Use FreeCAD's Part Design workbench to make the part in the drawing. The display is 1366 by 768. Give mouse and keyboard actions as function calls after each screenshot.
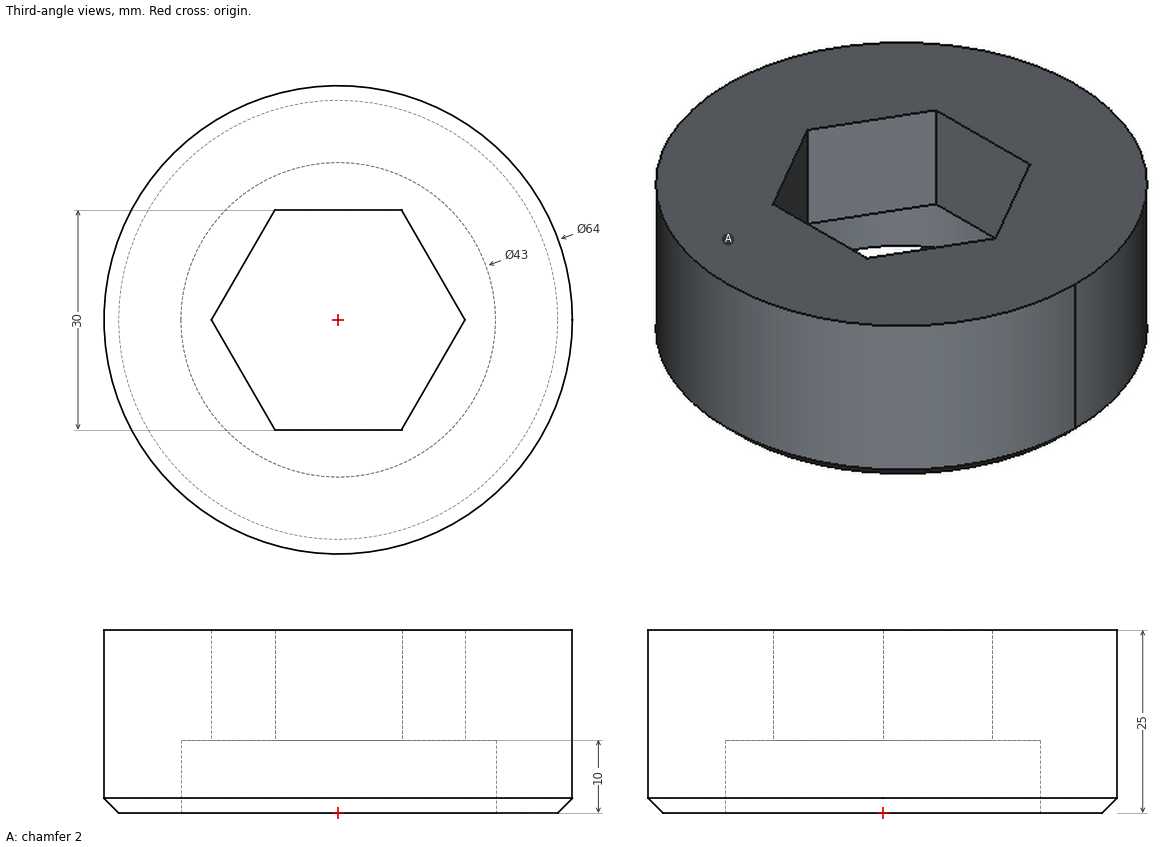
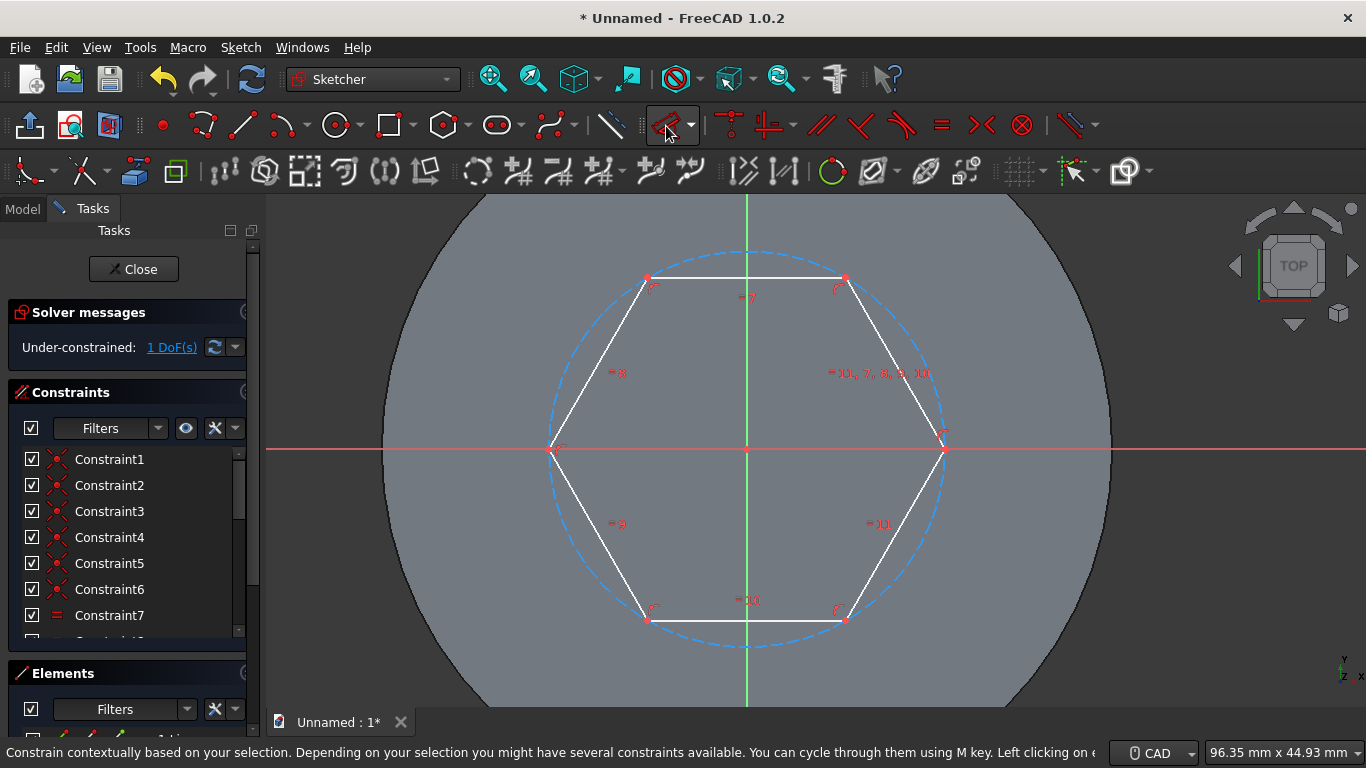
click(648, 621)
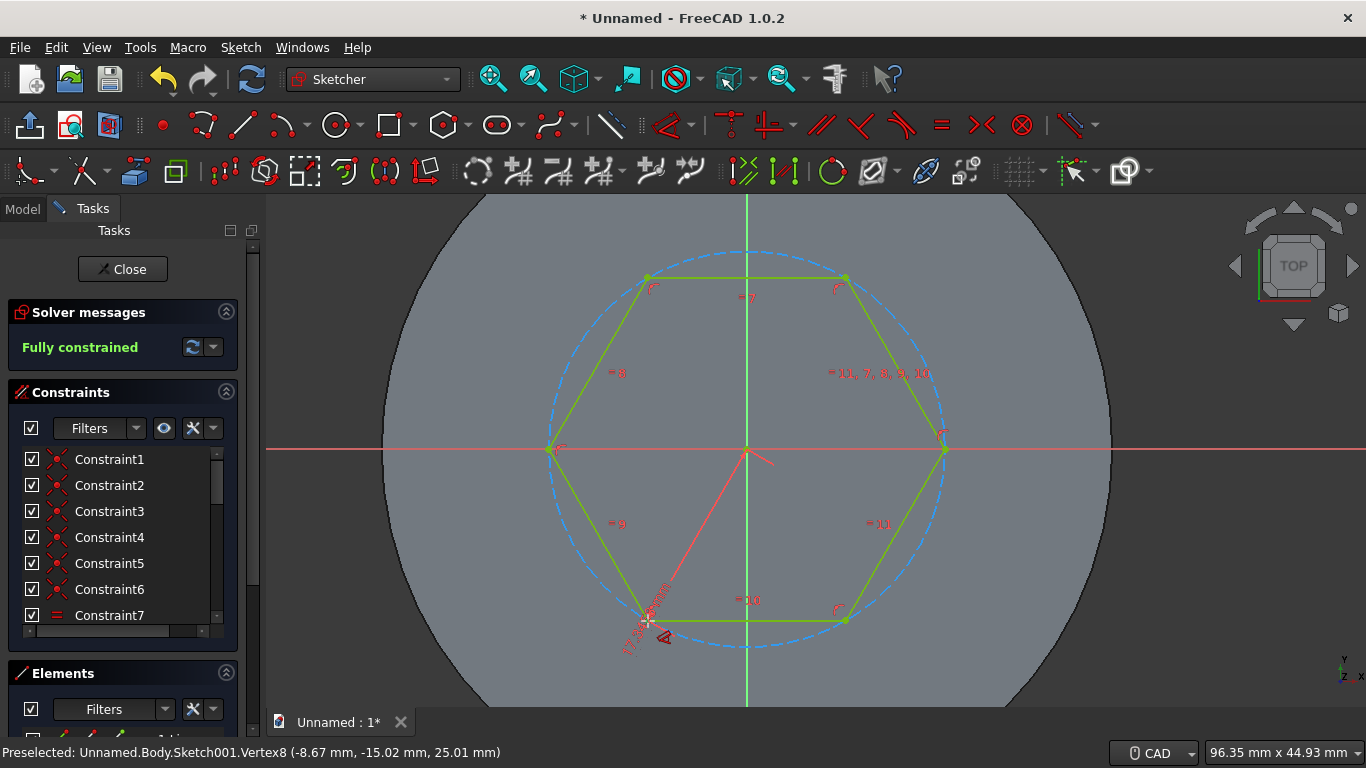
click(846, 278)
click(880, 370)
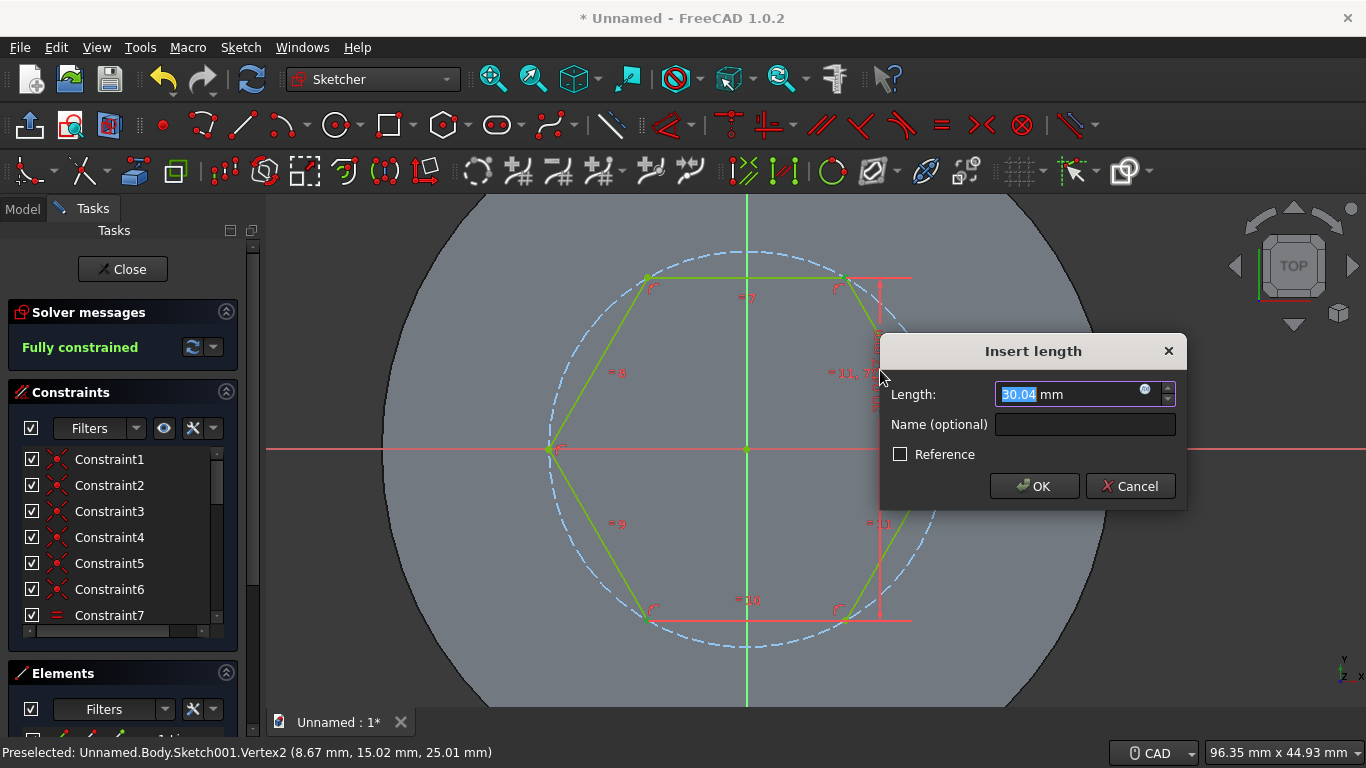
text(30)
key(Return)
key(Escape)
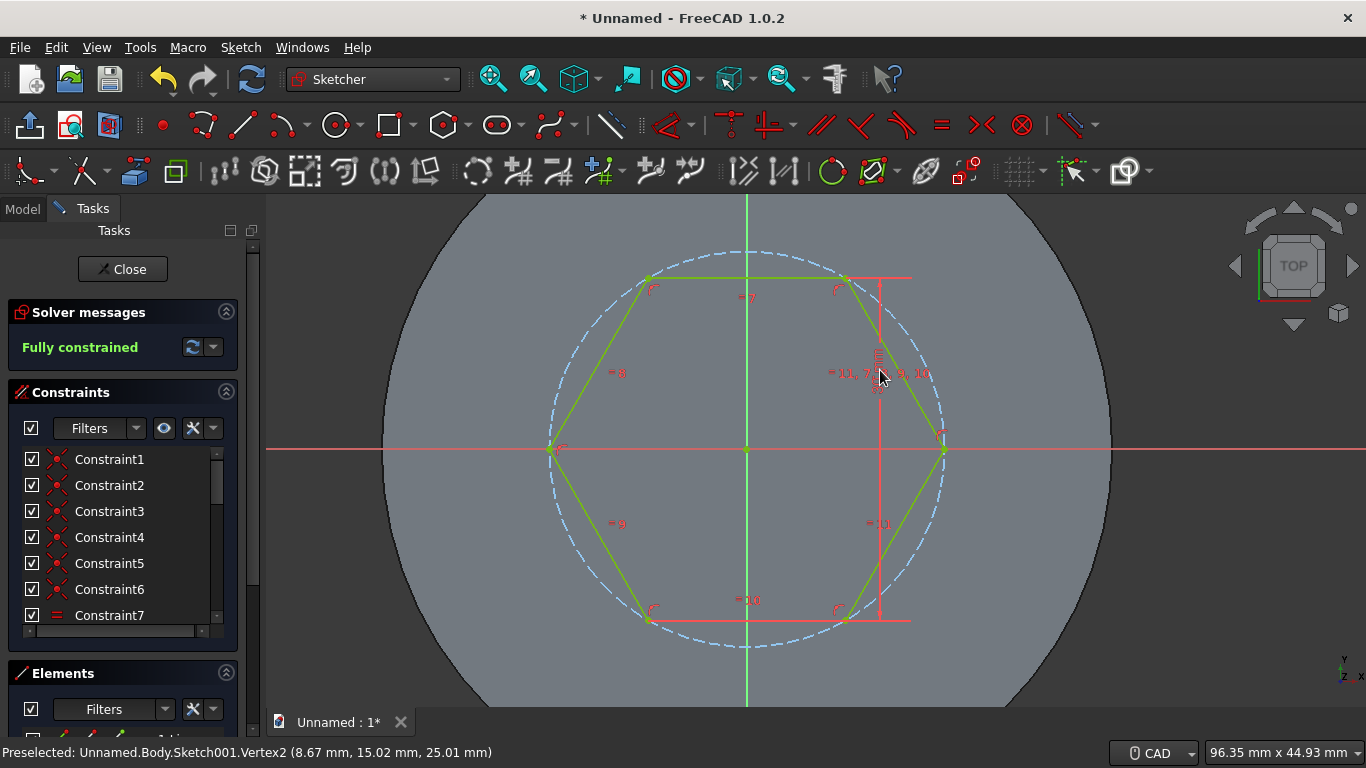
click(123, 269)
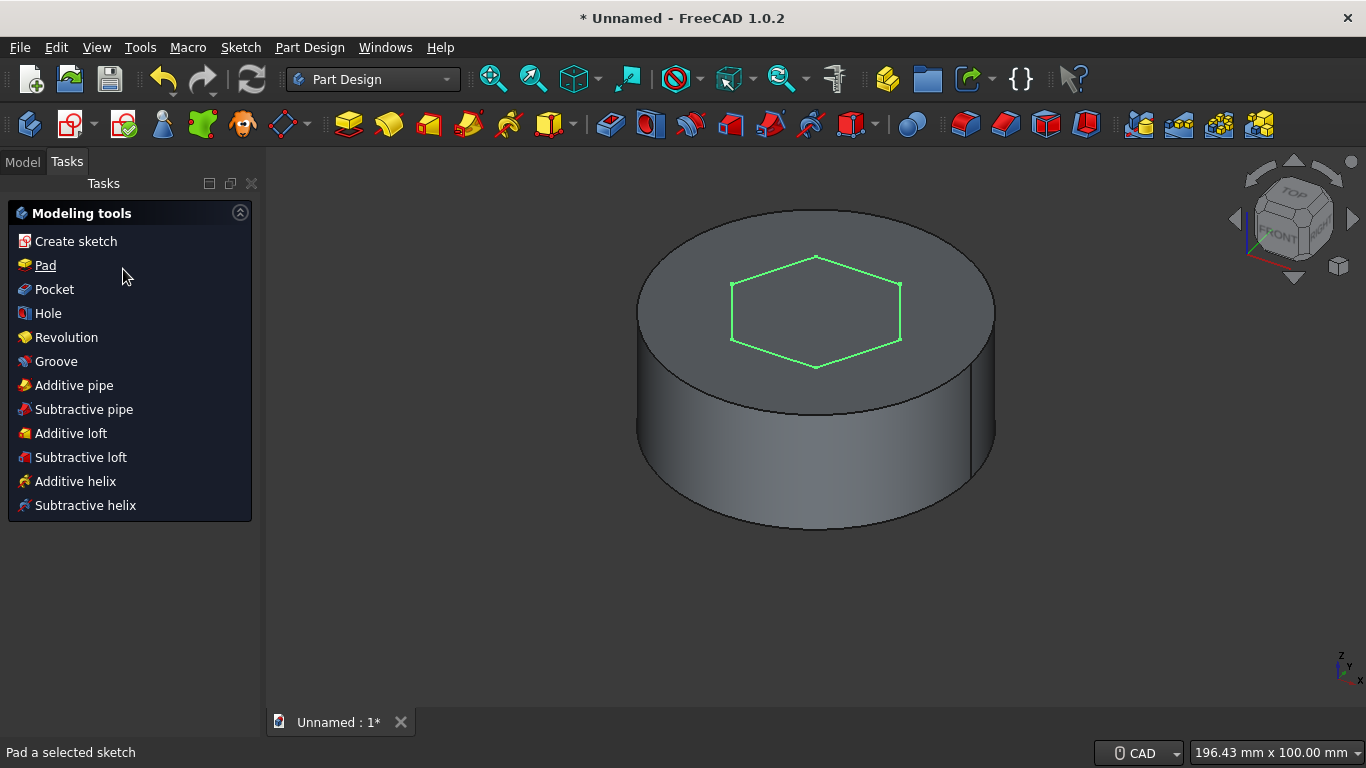
click(612, 124)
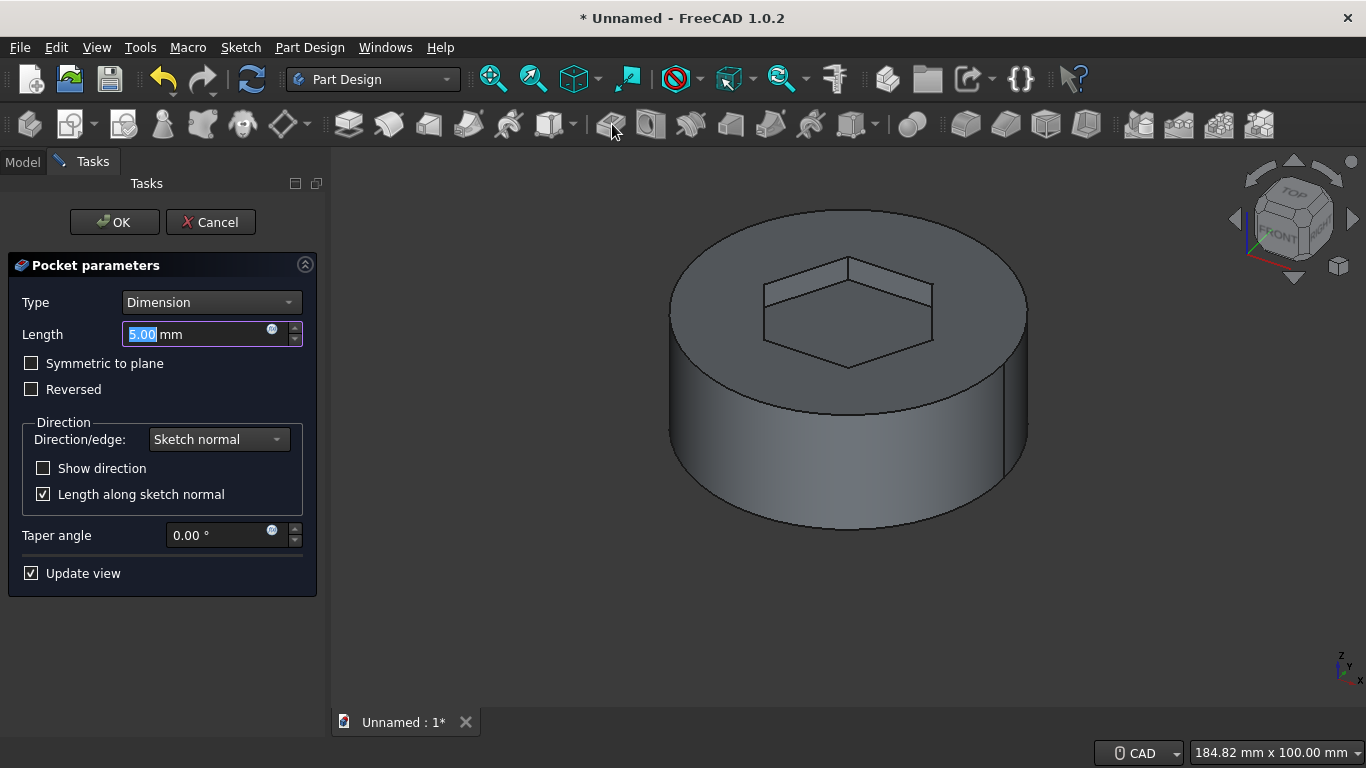
click(212, 302)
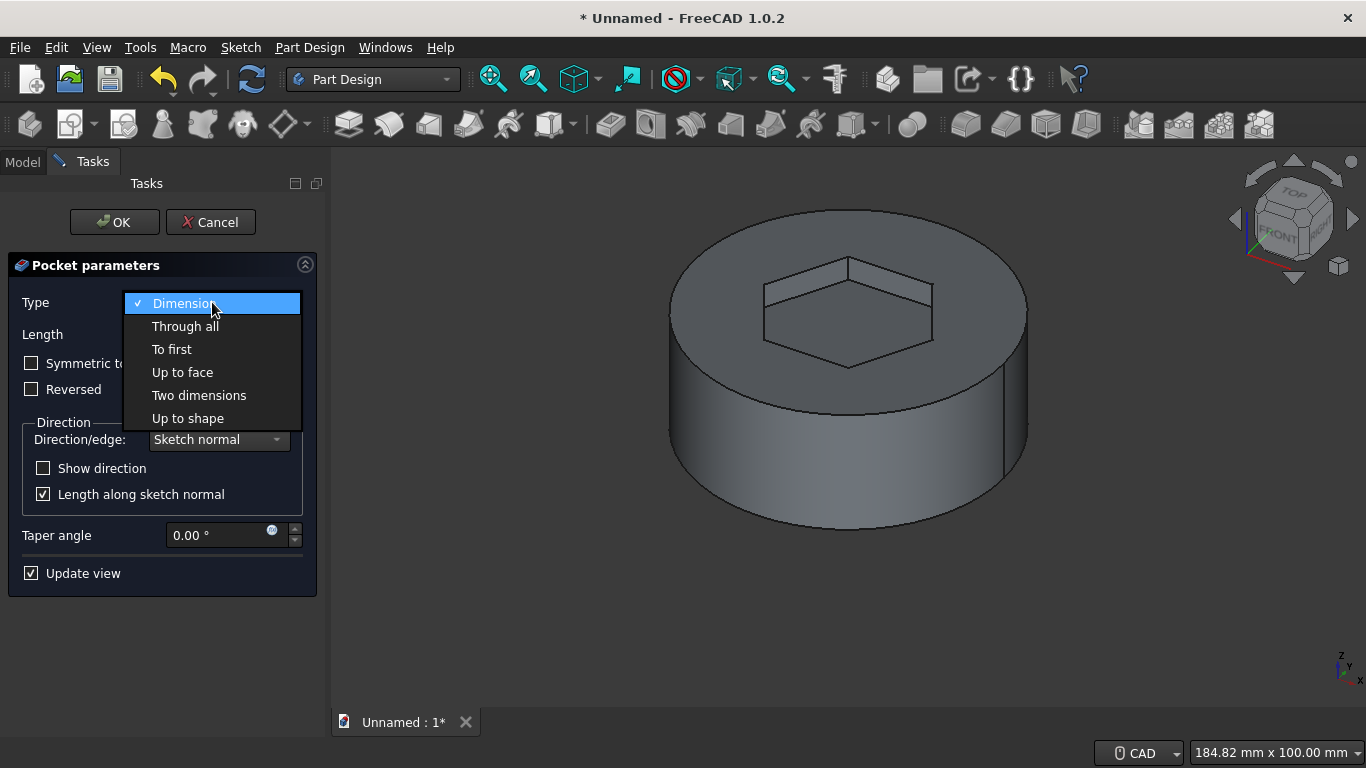
click(212, 326)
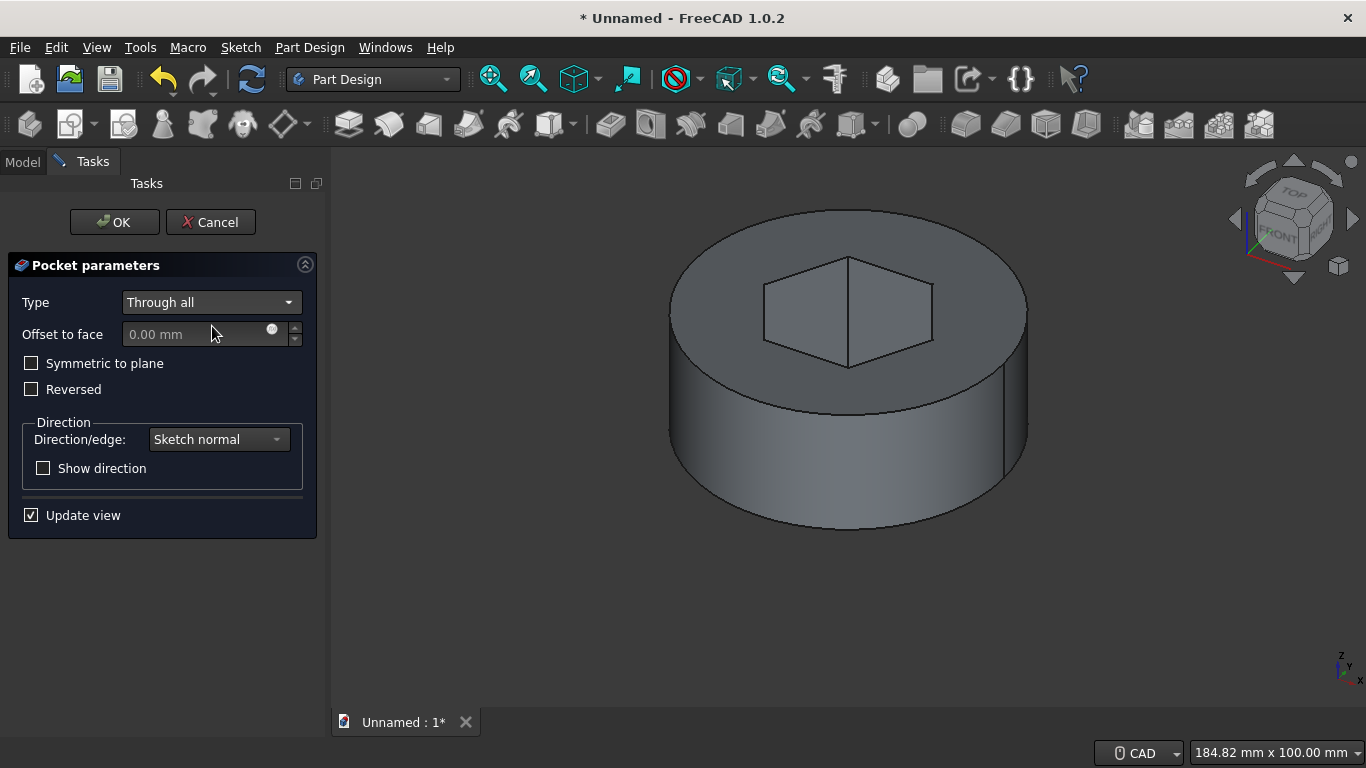
click(115, 222)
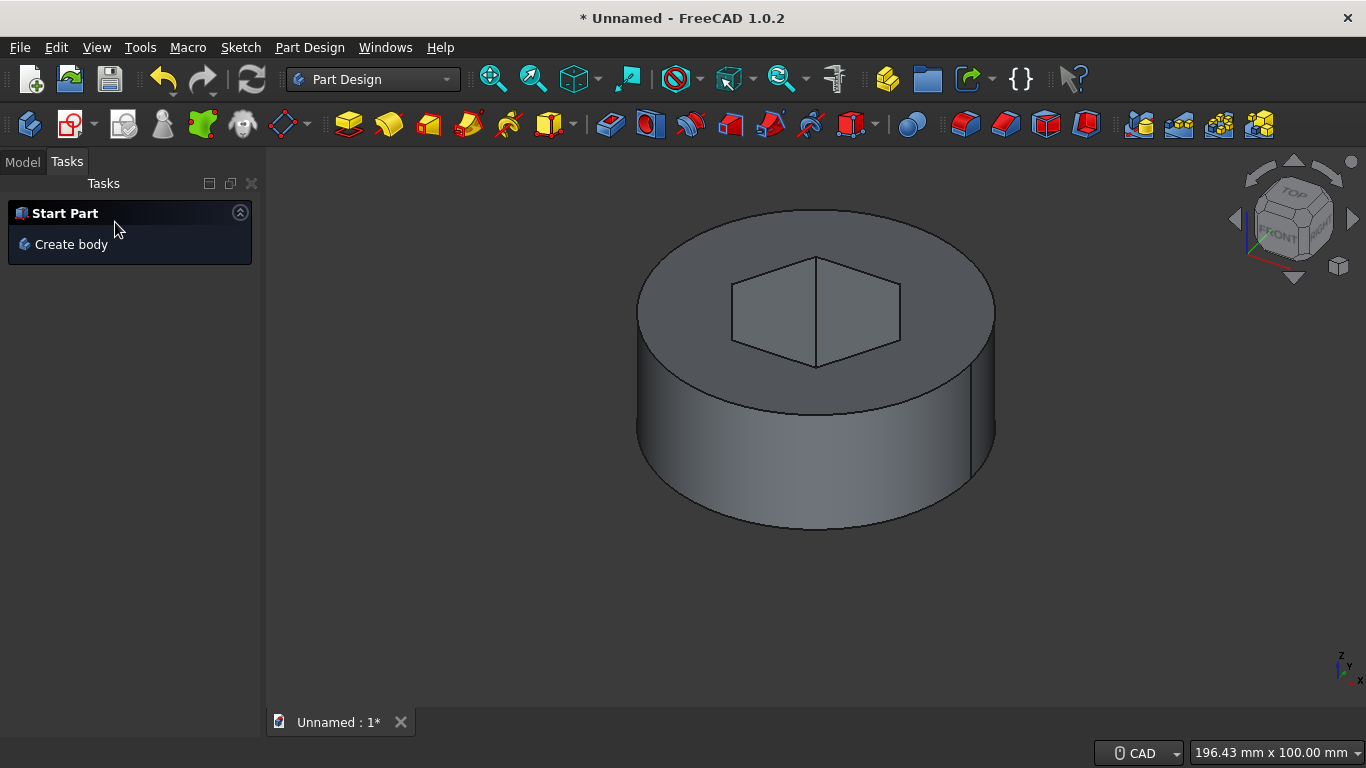
click(70, 124)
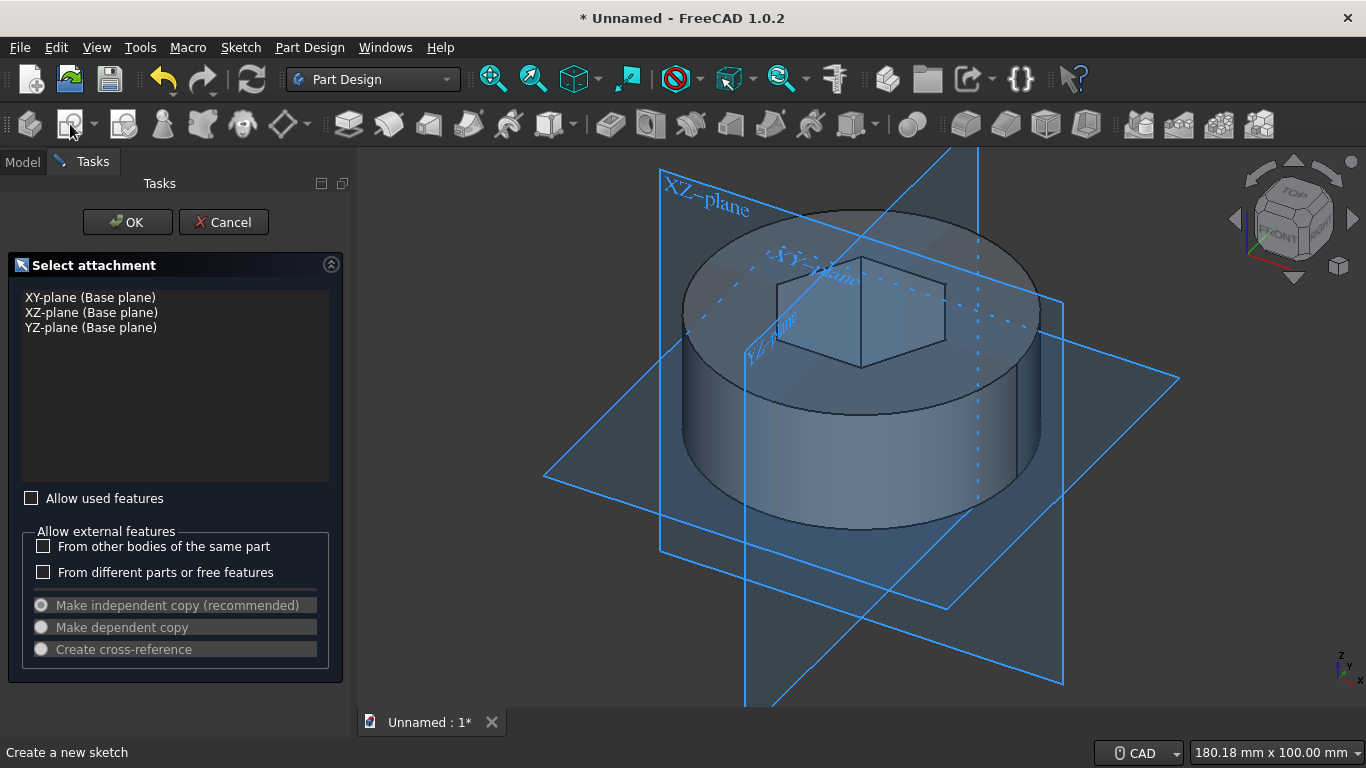
click(82, 298)